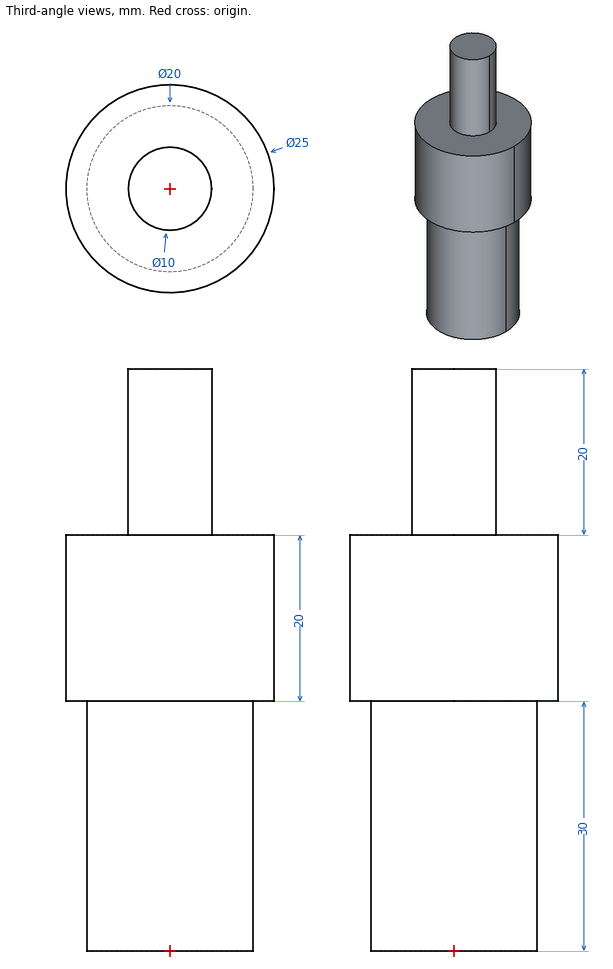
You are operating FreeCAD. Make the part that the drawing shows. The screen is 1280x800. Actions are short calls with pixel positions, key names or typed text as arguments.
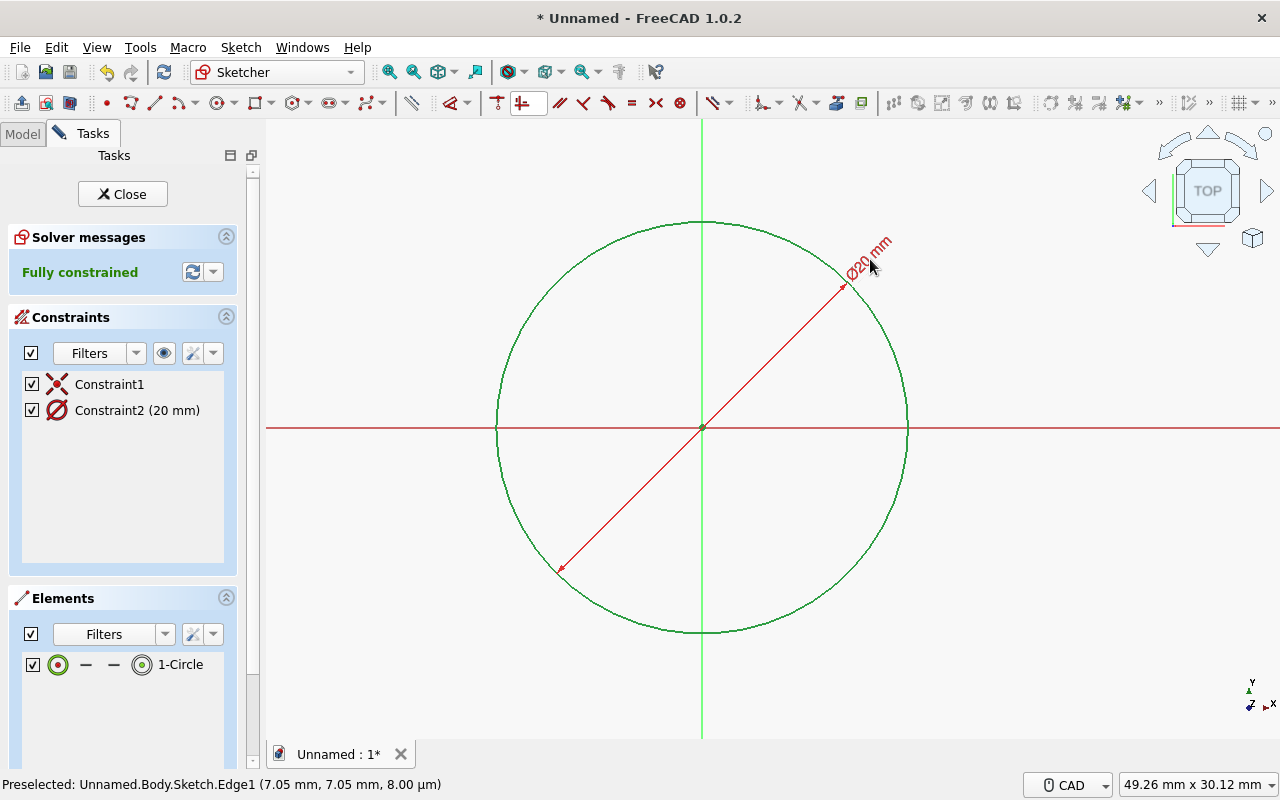
click(123, 194)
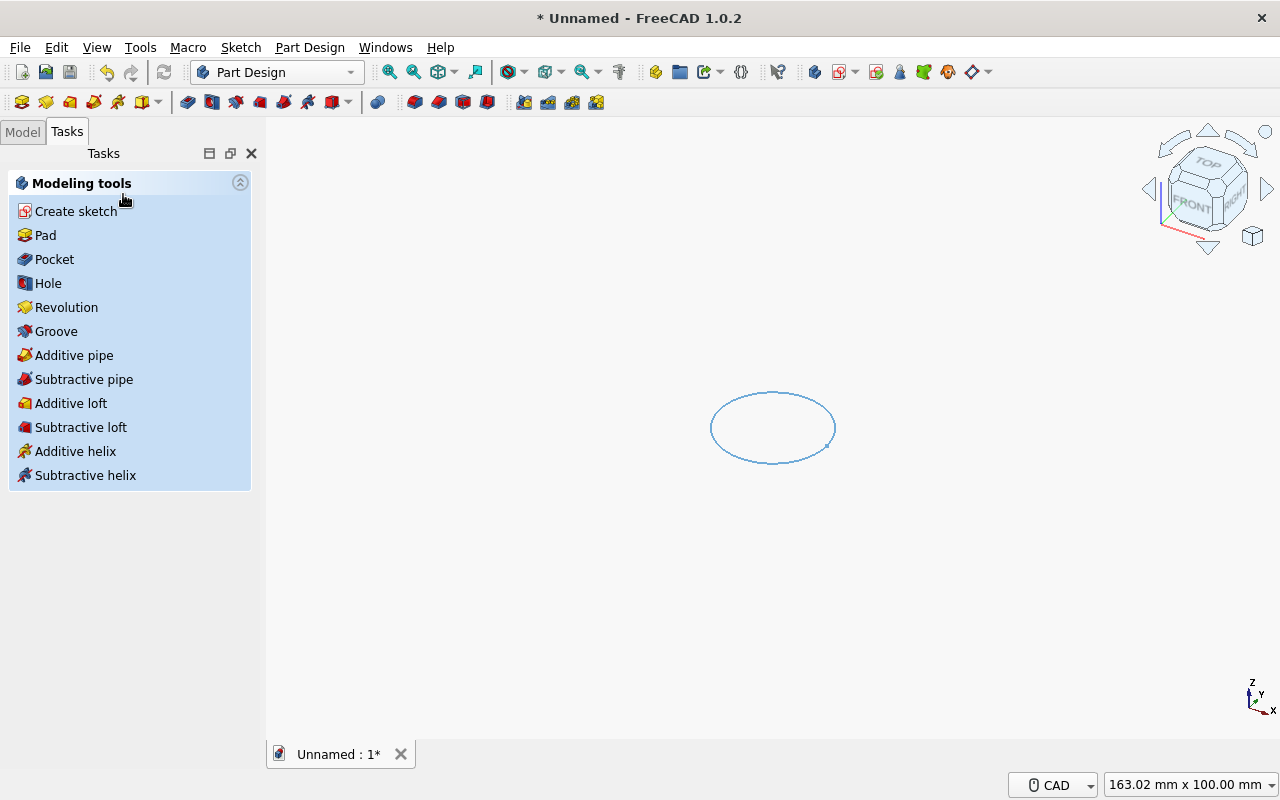
click(22, 102)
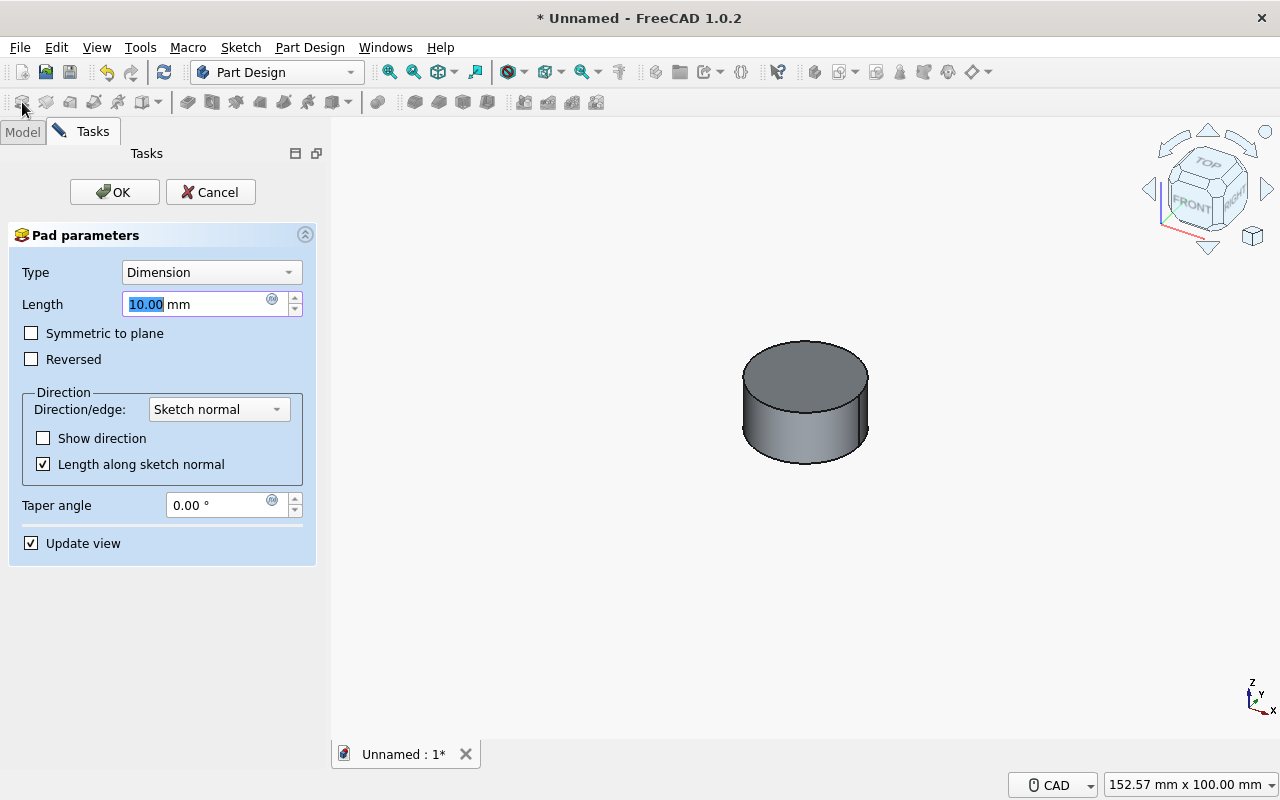
text(30)
key(Tab)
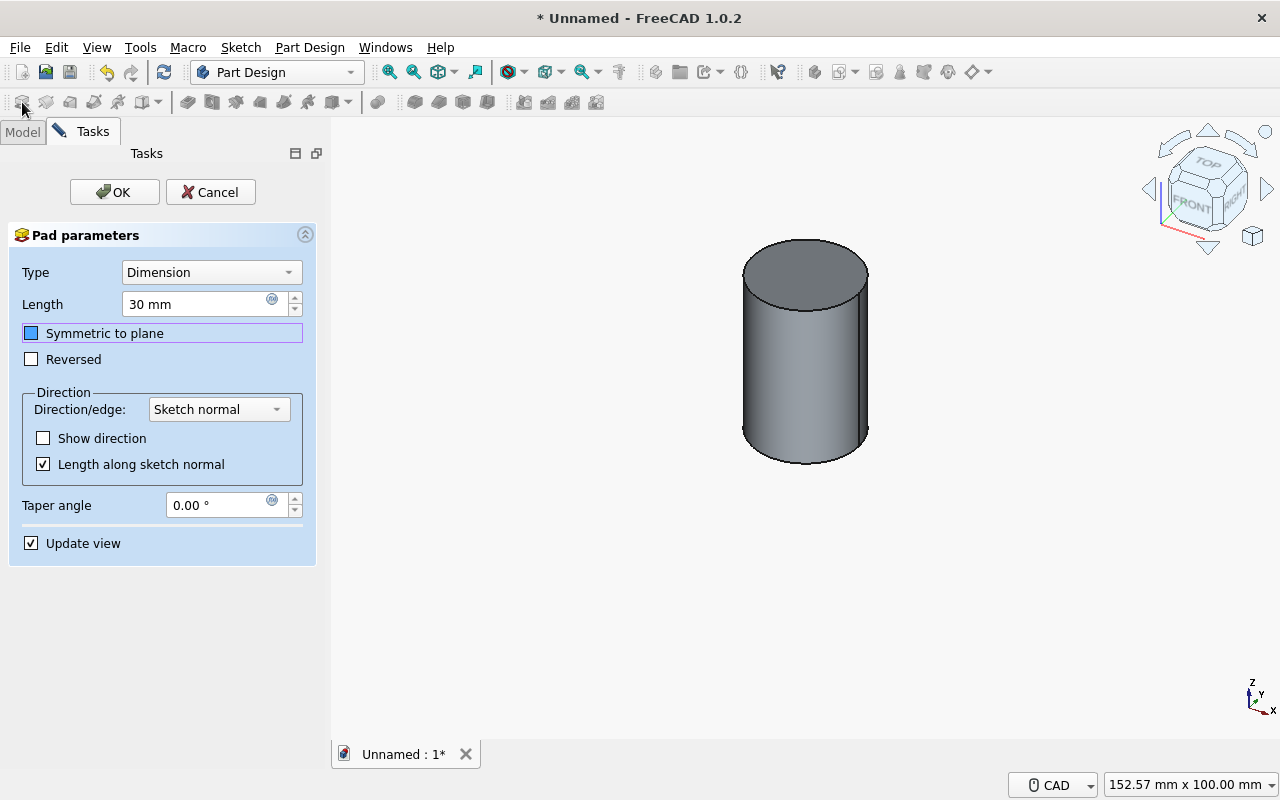
click(115, 192)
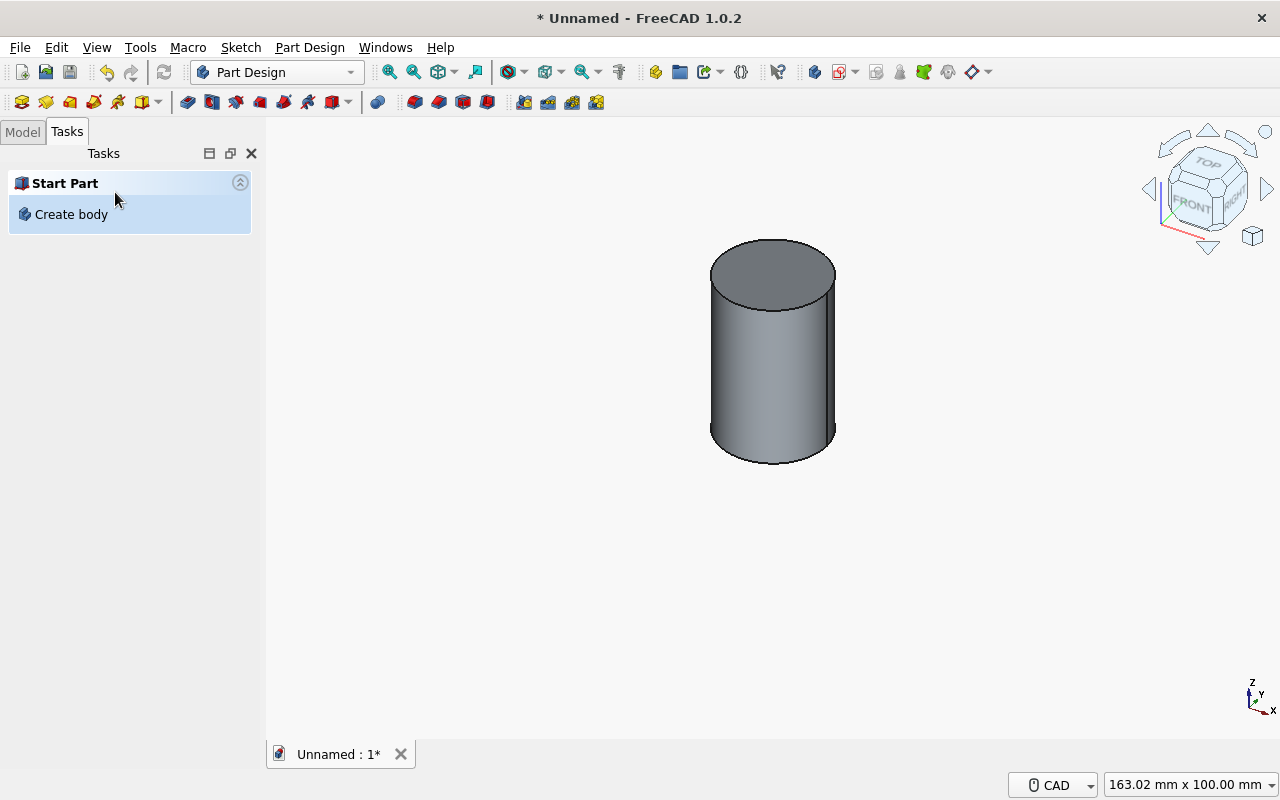
click(390, 72)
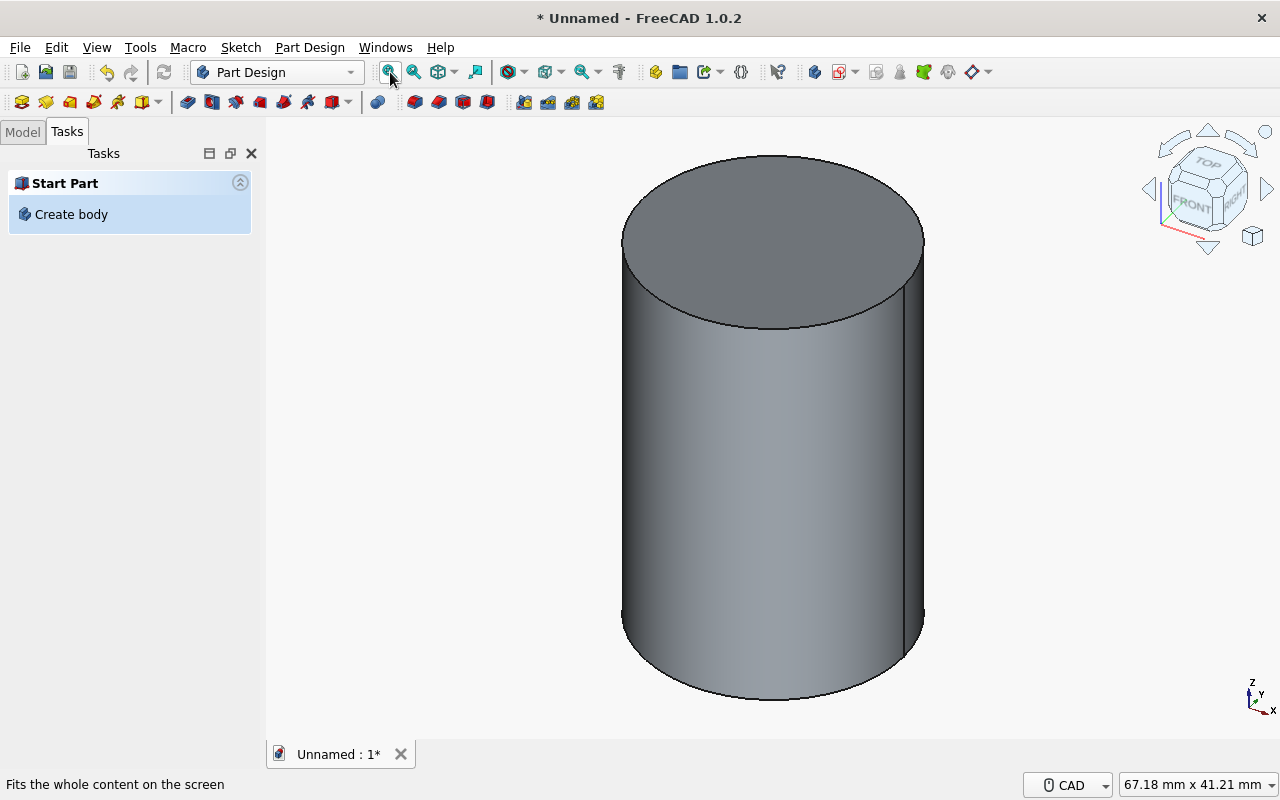
click(773, 242)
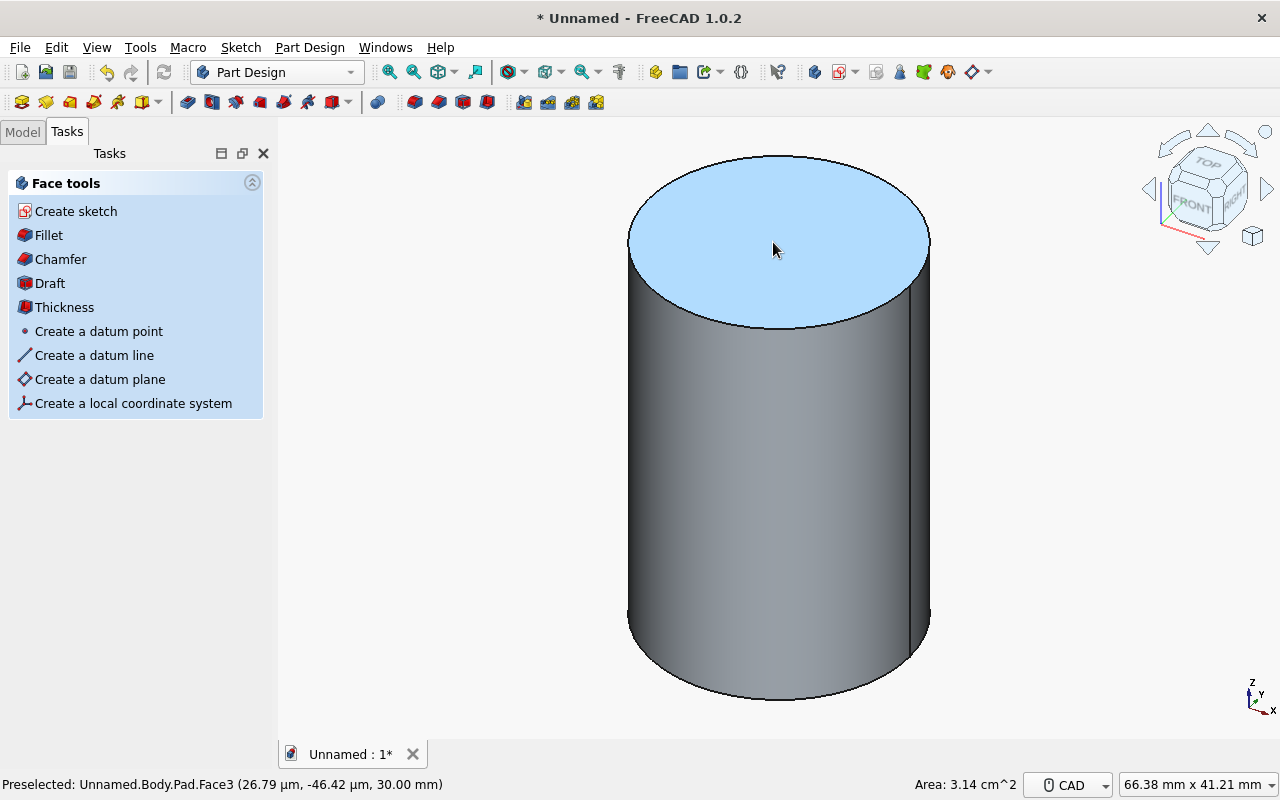
click(840, 72)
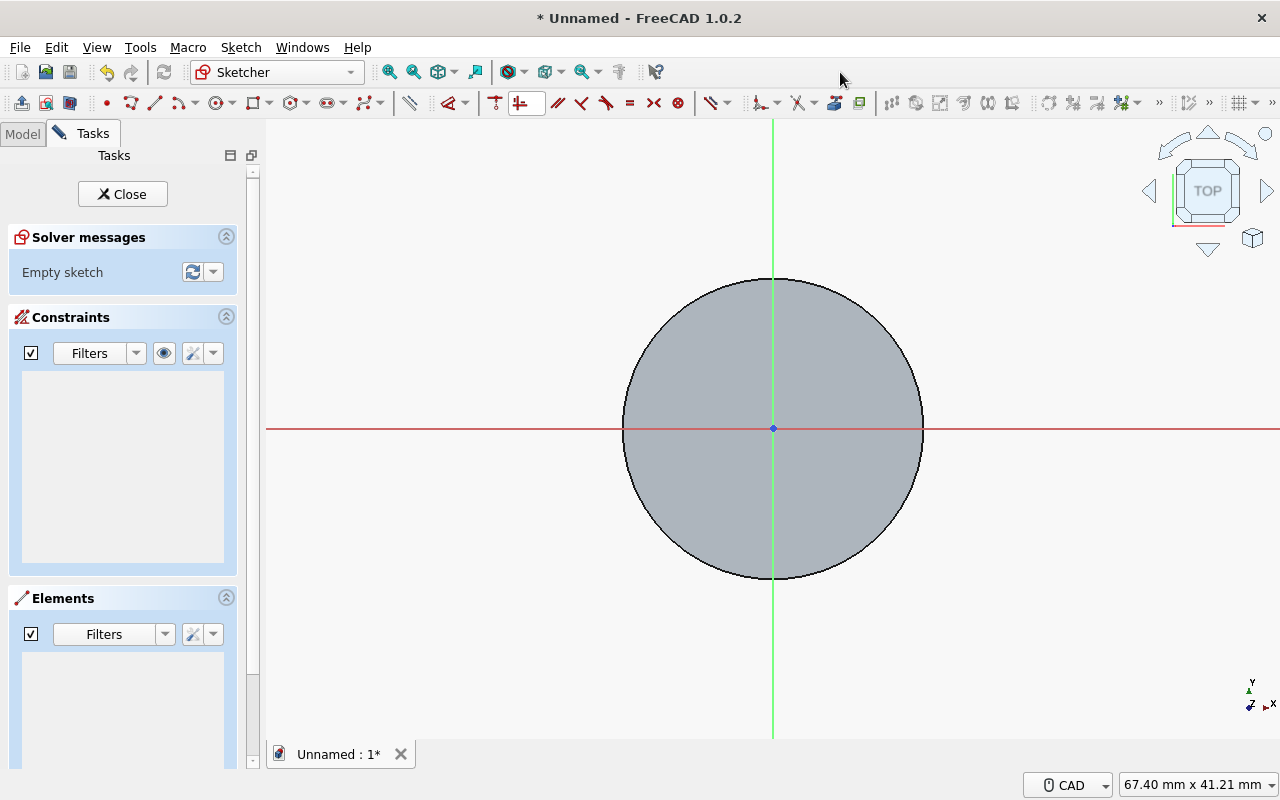
key(g)
key(c)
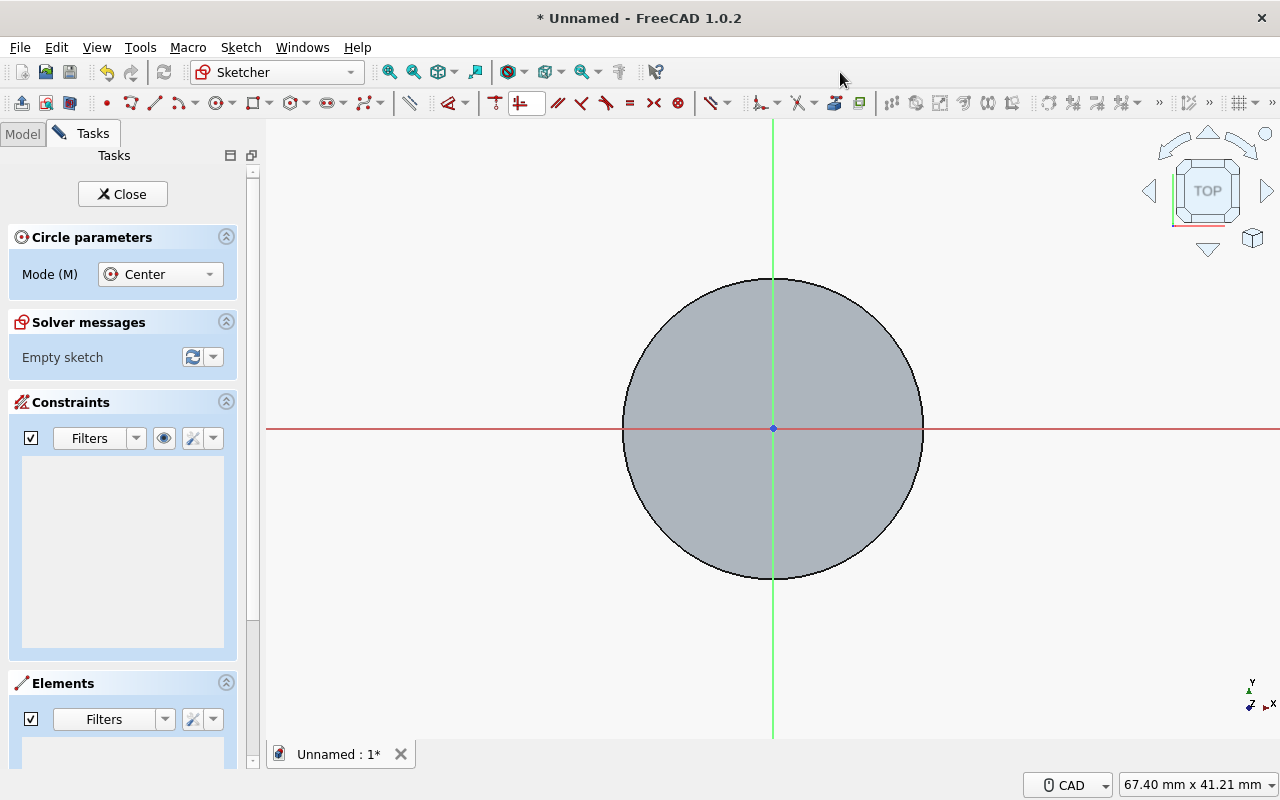
click(773, 429)
click(906, 296)
key(Escape)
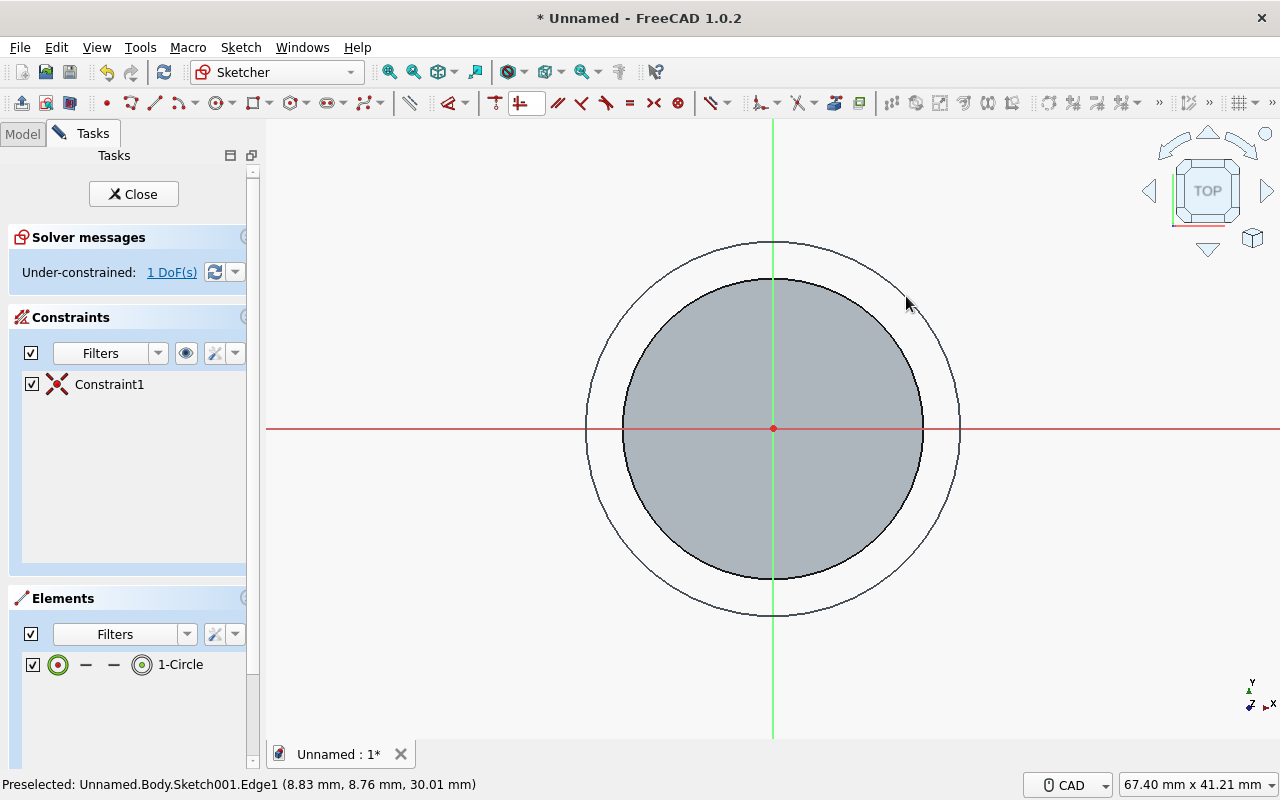
key(d)